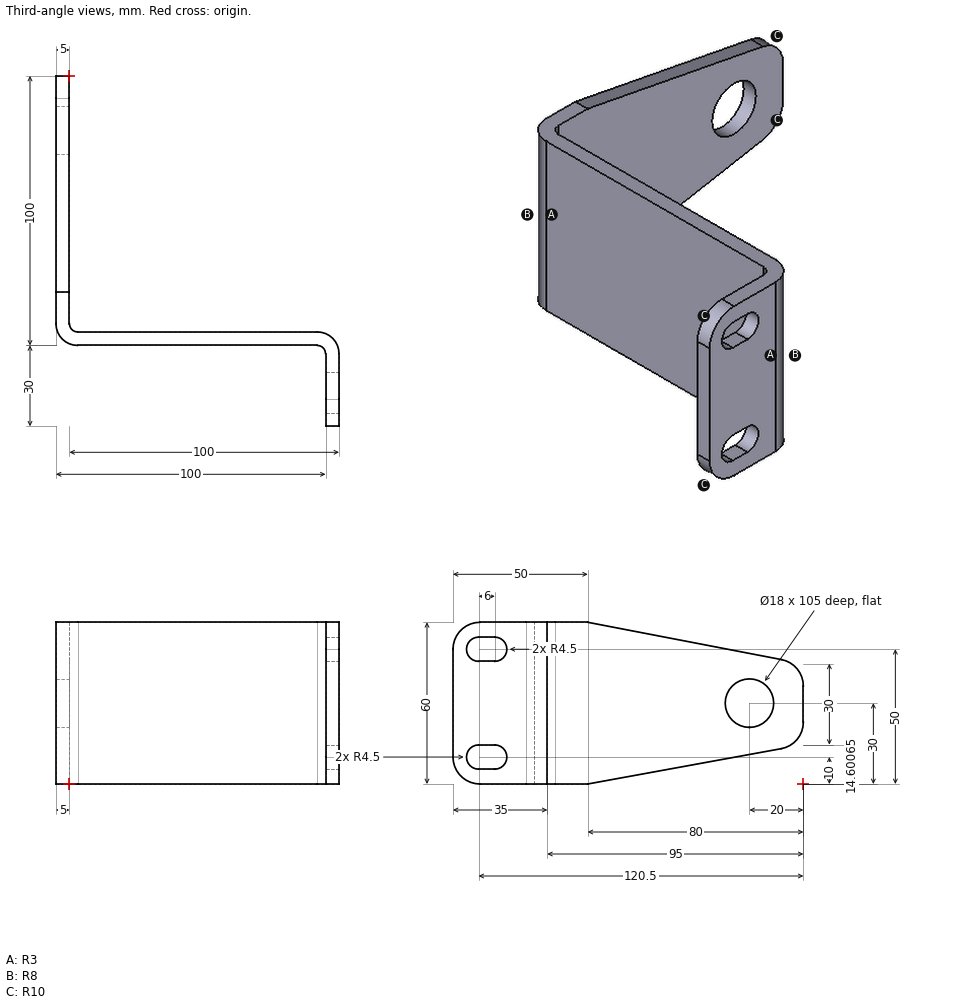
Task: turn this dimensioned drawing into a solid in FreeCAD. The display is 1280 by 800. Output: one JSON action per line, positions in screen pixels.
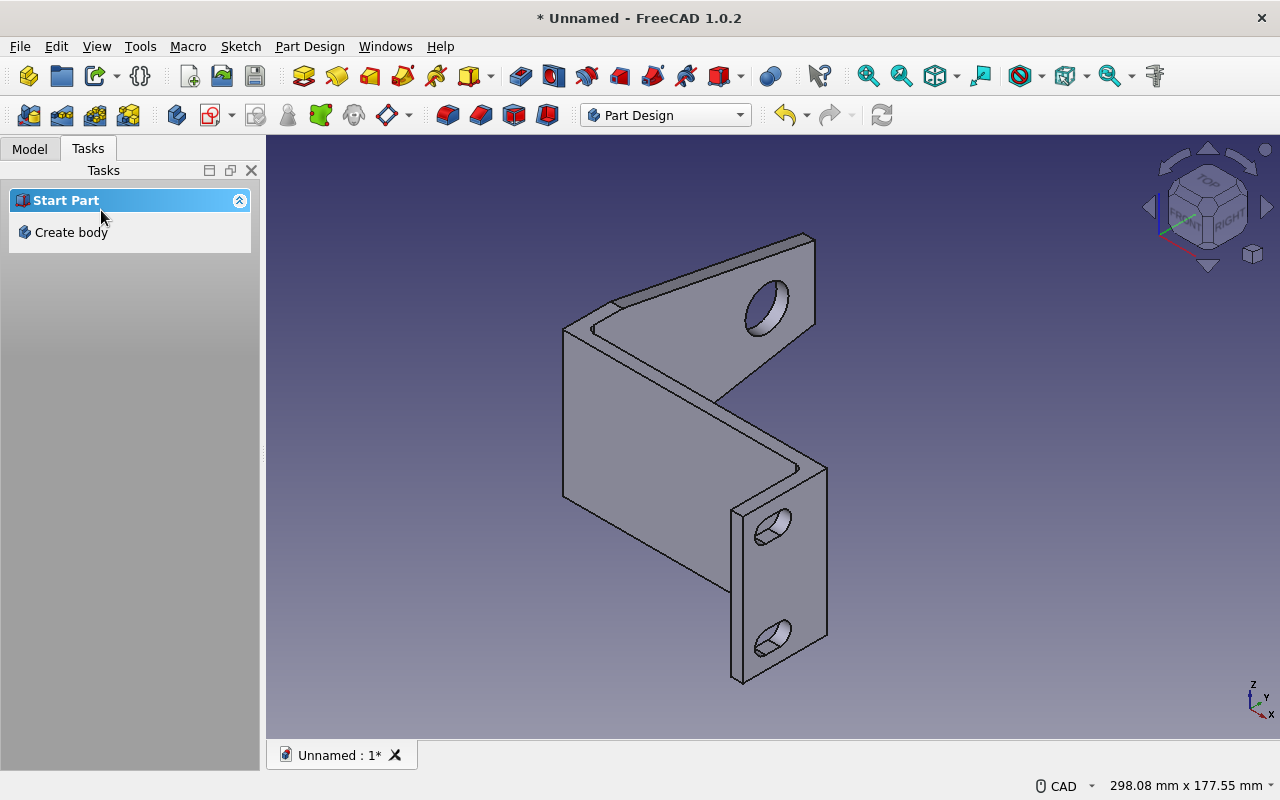
{"action": "key", "text": "1"}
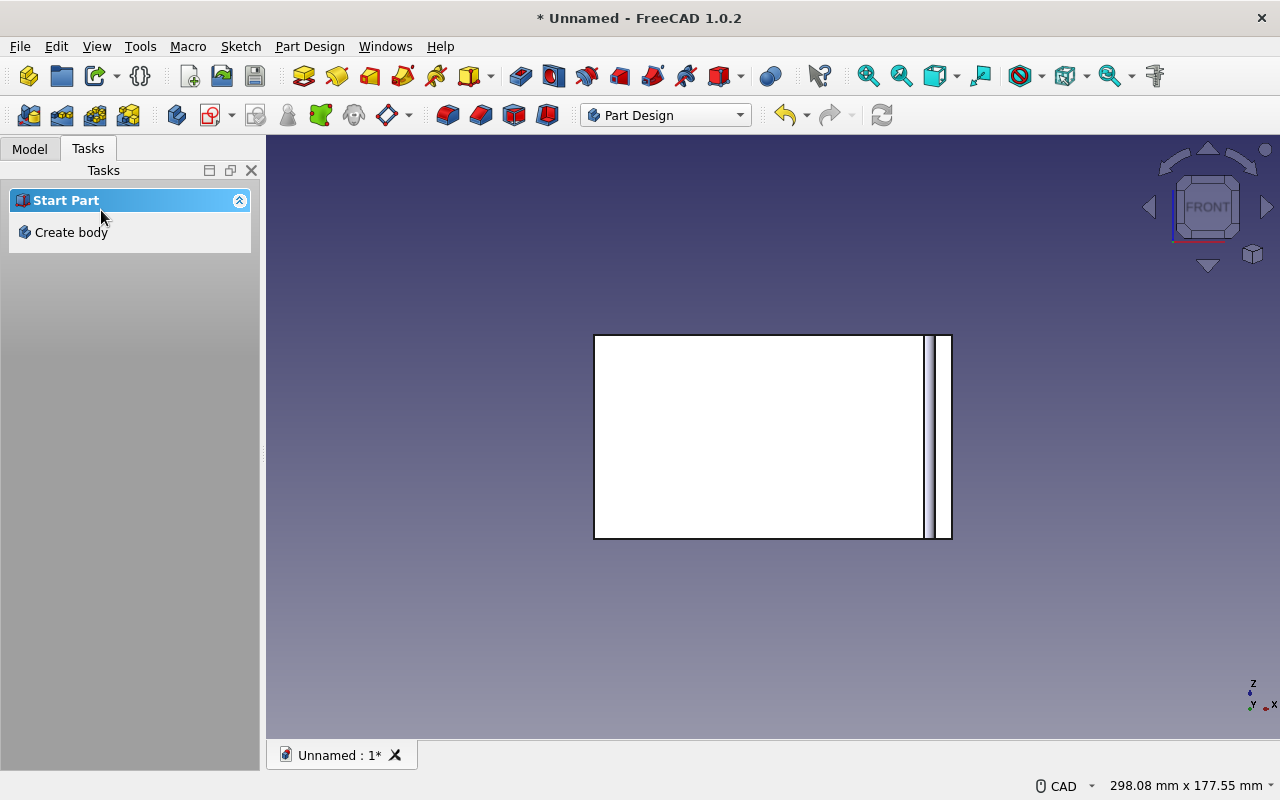
{"action": "left_click", "coordinate": [869, 76]}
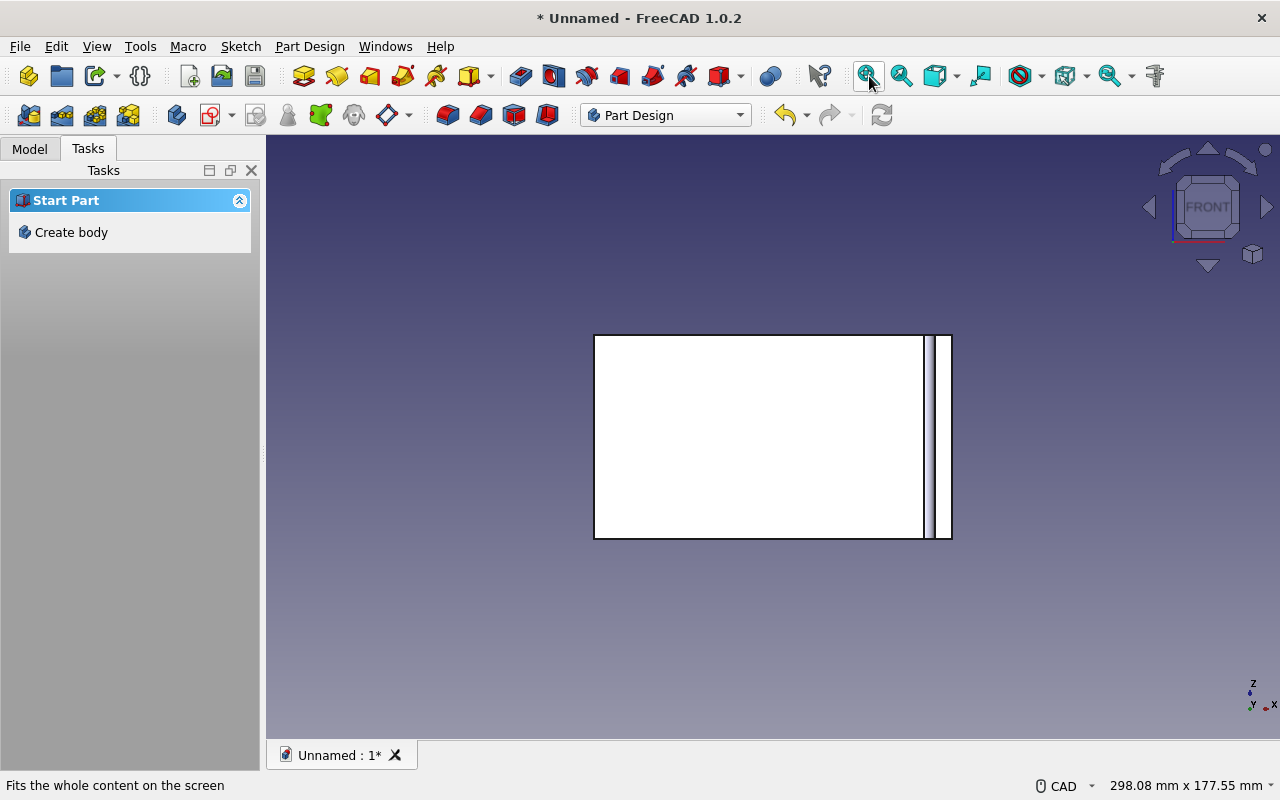
{"action": "left_click", "coordinate": [594, 436]}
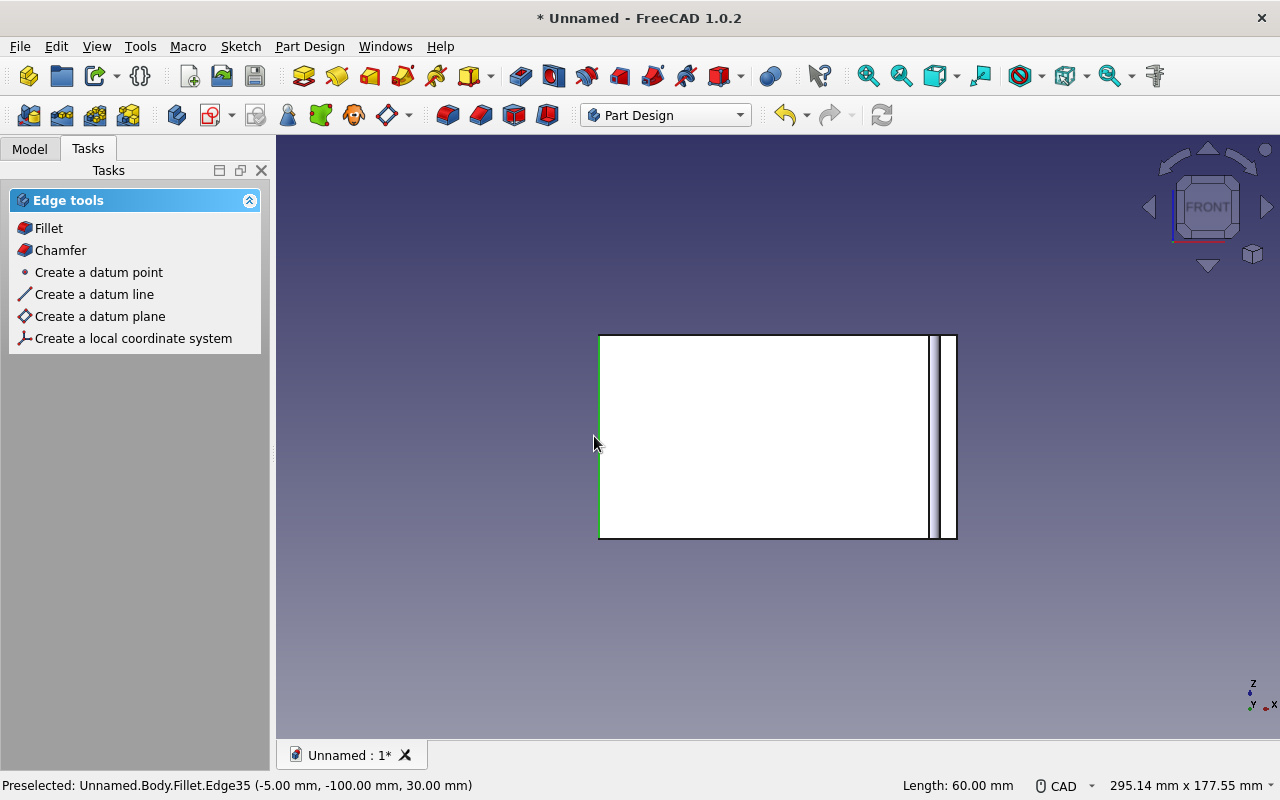
{"action": "key", "text": "3"}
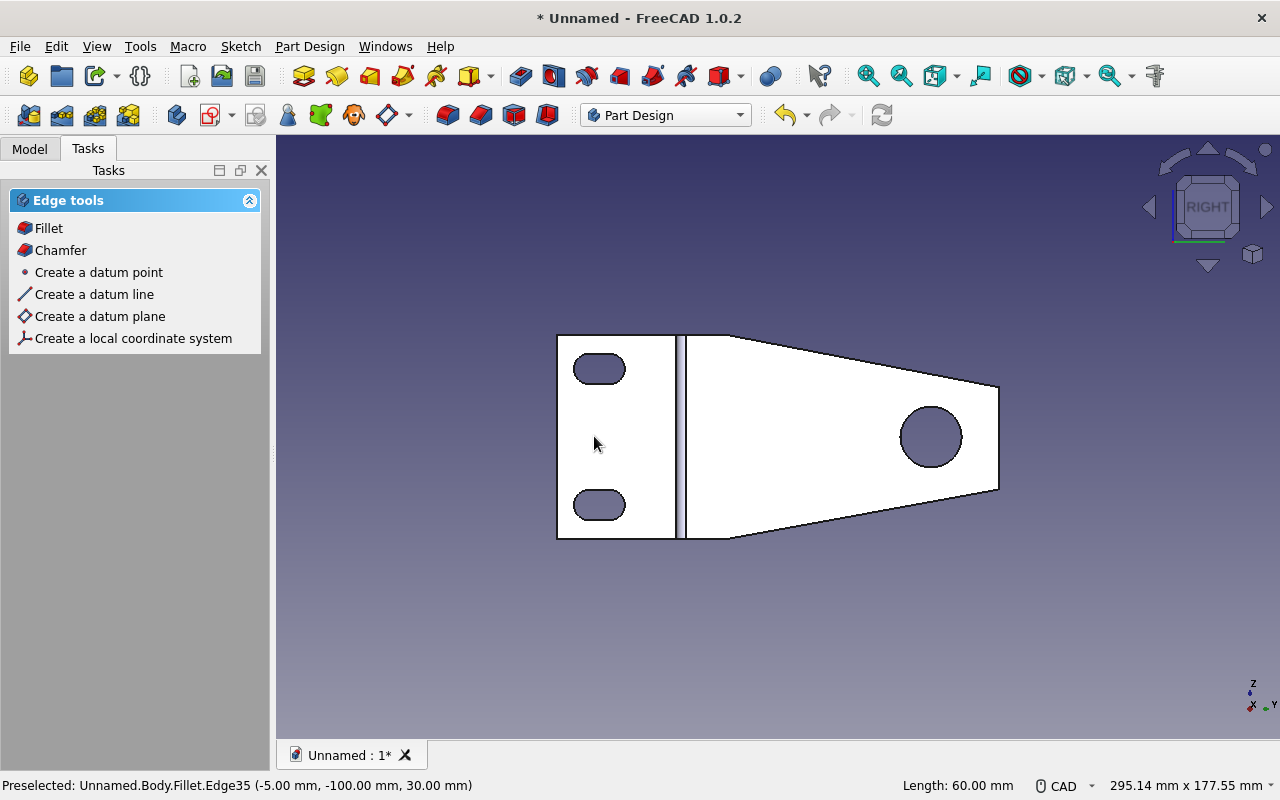
{"action": "left_click", "coordinate": [869, 76]}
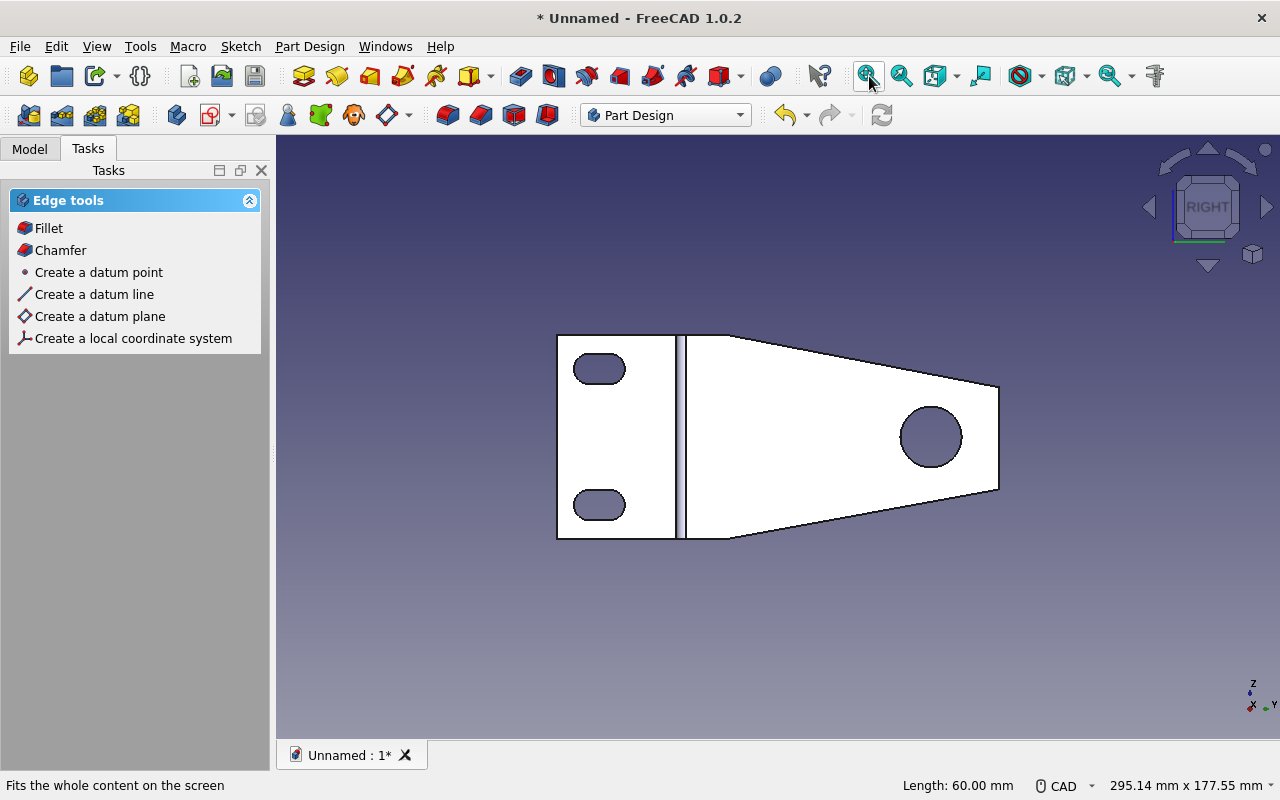
{"action": "left_click", "coordinate": [676, 436], "text": "ctrl"}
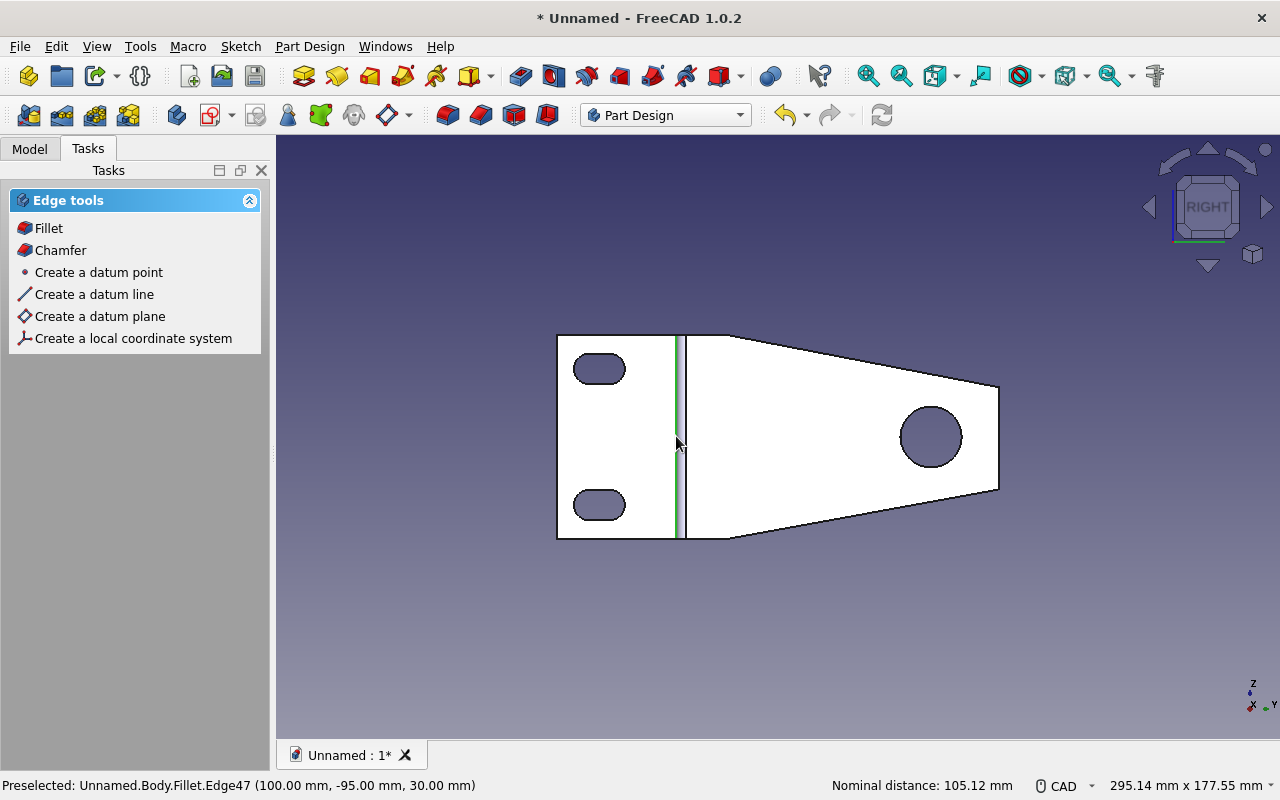
{"action": "left_click", "coordinate": [448, 116]}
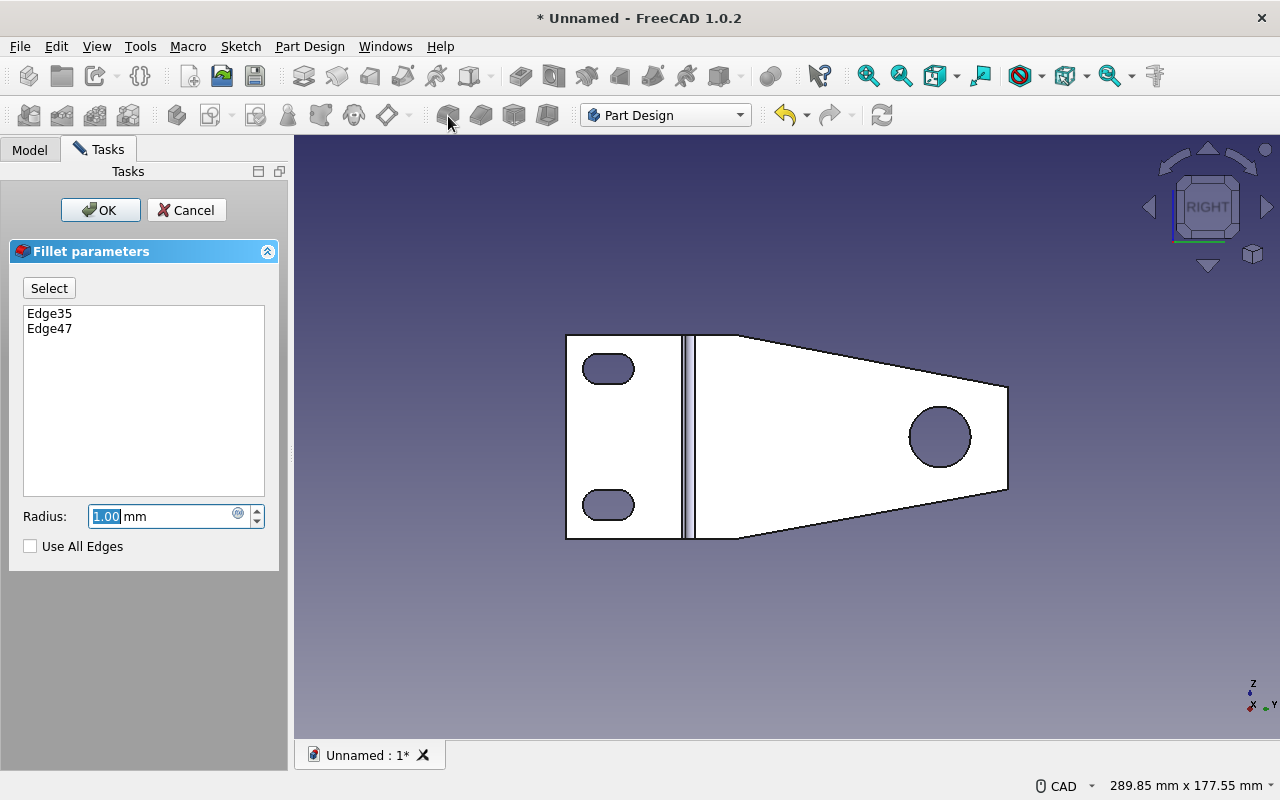
{"action": "type", "text": "8"}
{"action": "key", "text": "Tab"}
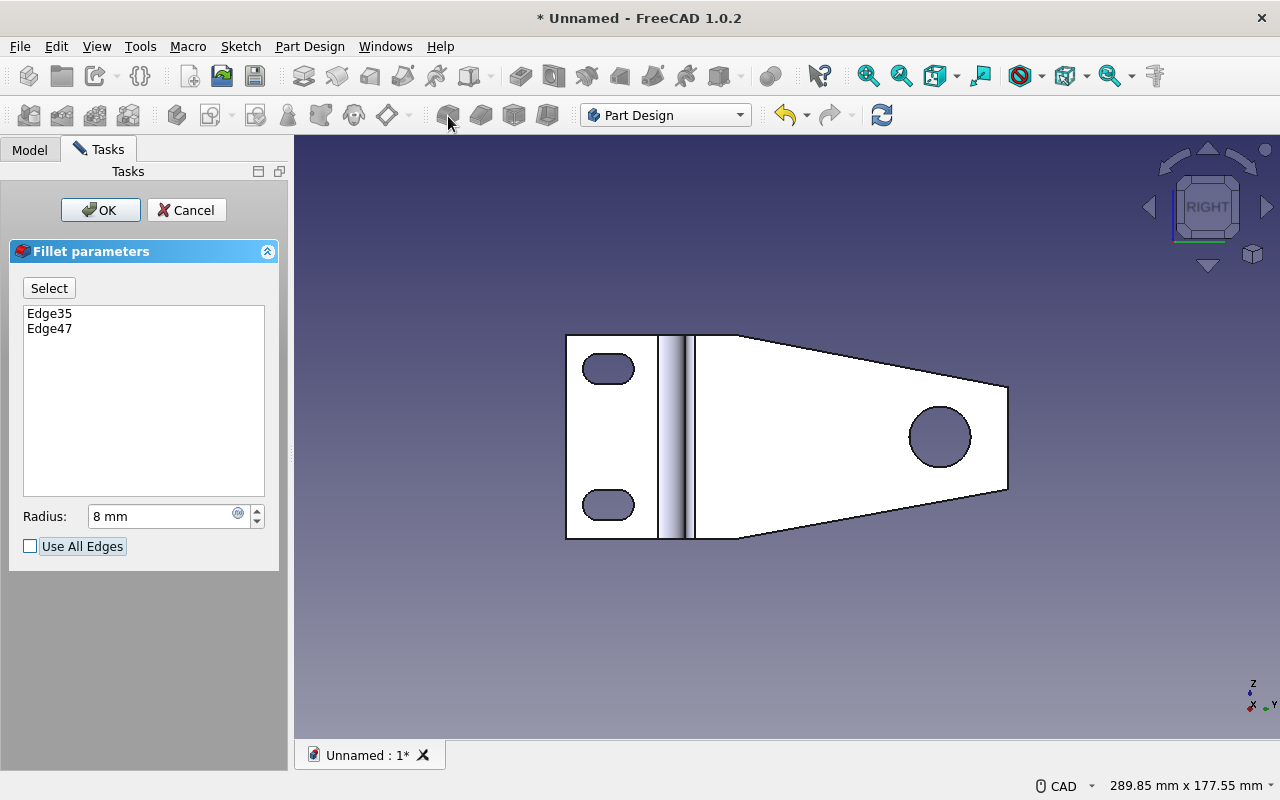
{"action": "left_click", "coordinate": [101, 210]}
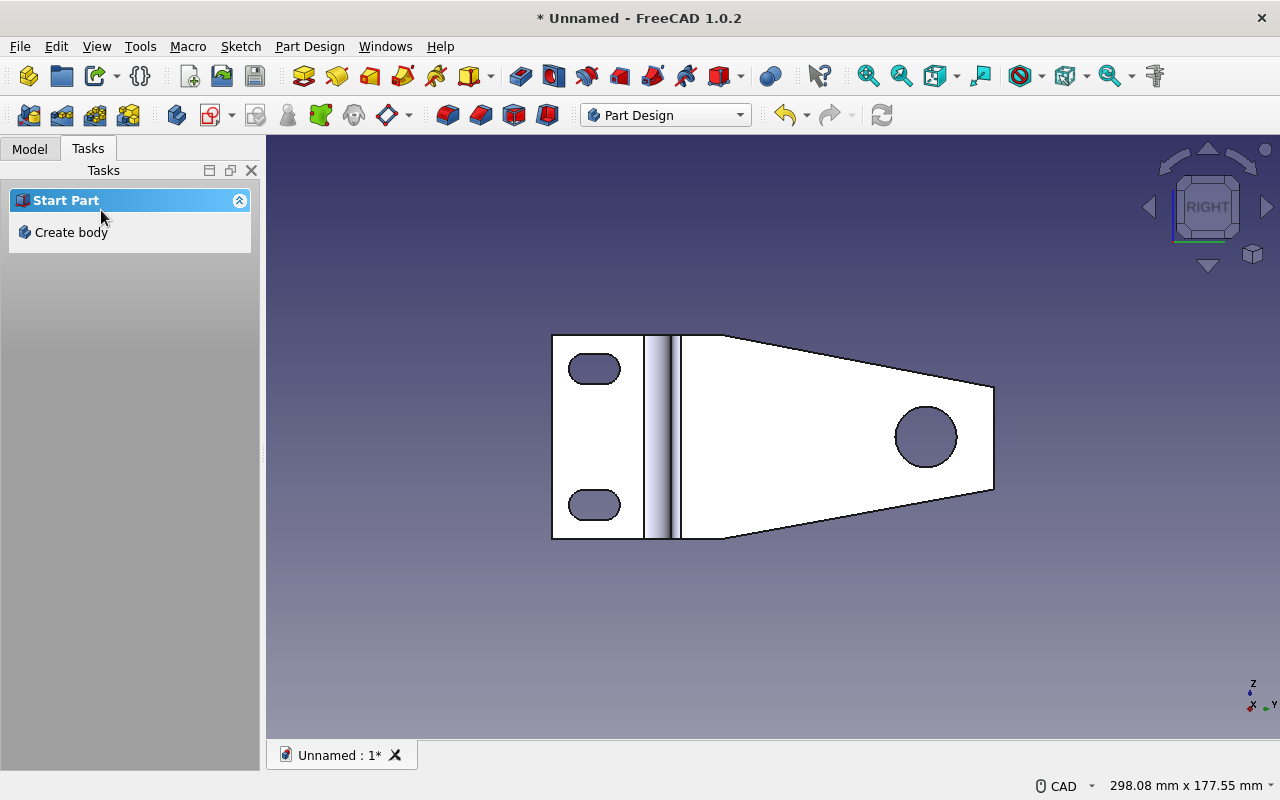
{"action": "left_click", "coordinate": [869, 76]}